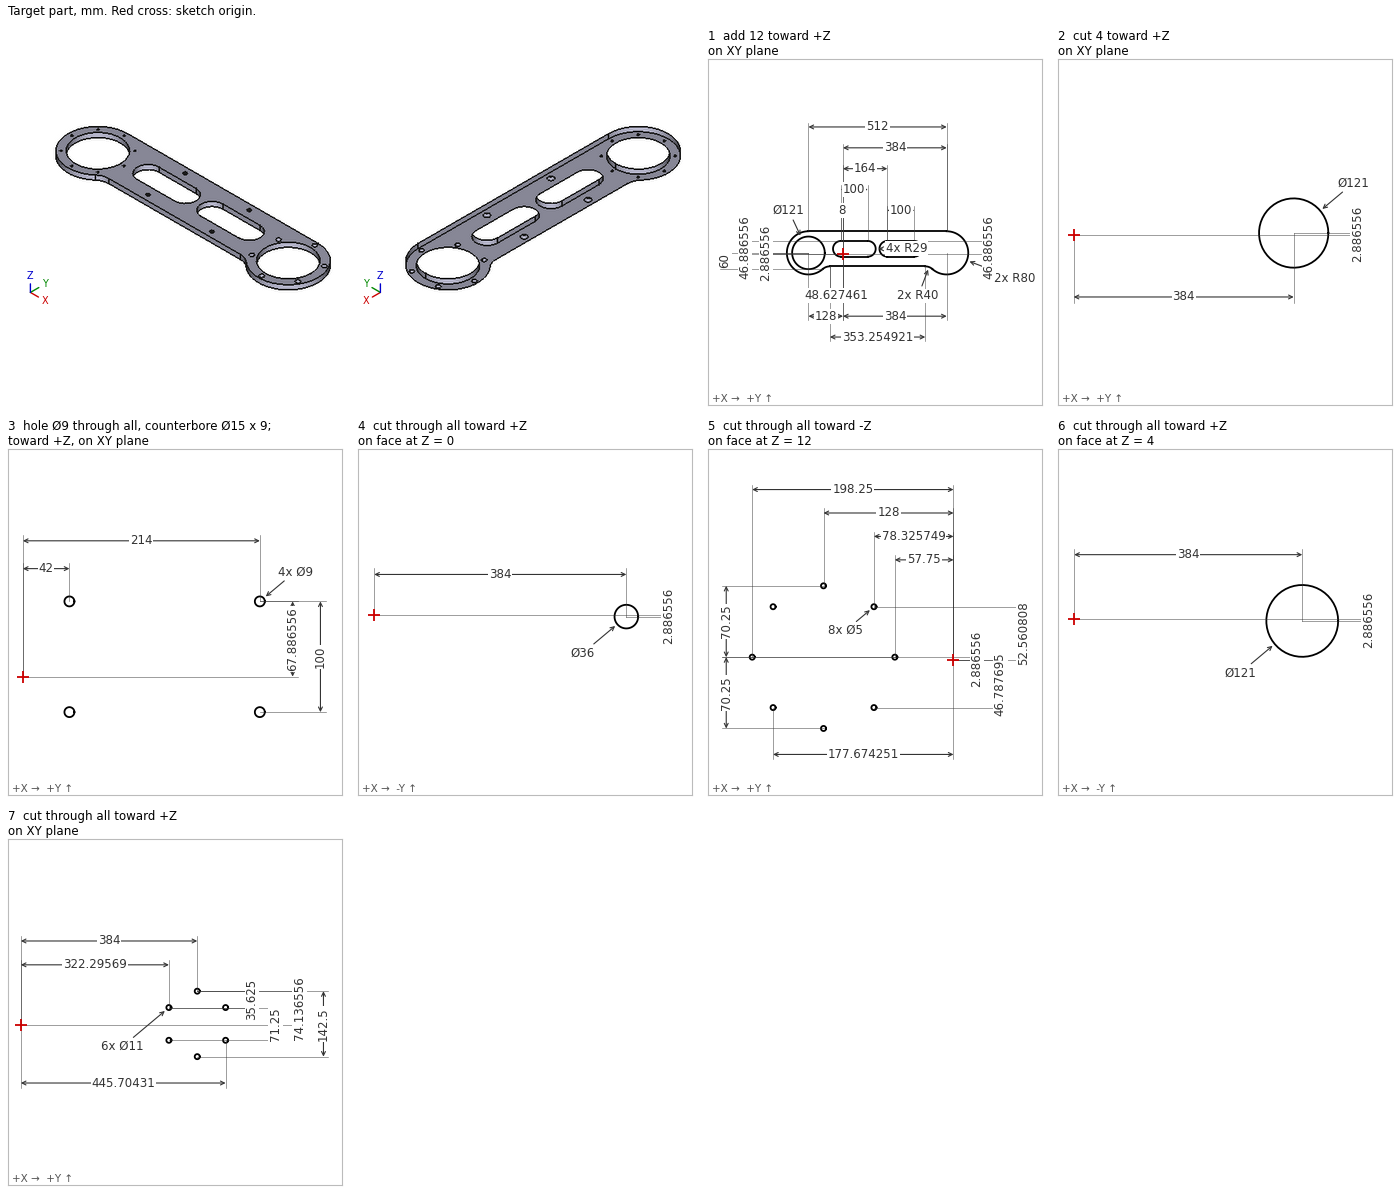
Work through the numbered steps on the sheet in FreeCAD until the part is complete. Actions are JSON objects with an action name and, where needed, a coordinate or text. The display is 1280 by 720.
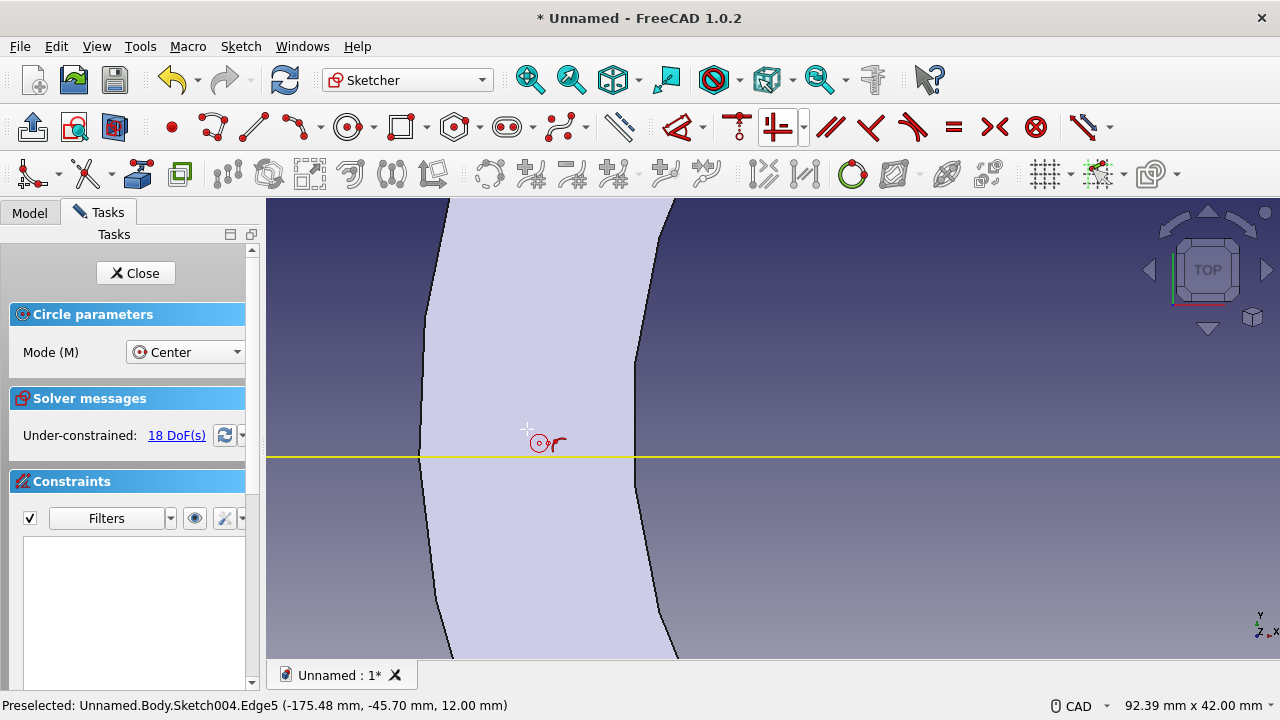
{"action": "left_click", "coordinate": [525, 425]}
{"action": "left_click", "coordinate": [545, 406]}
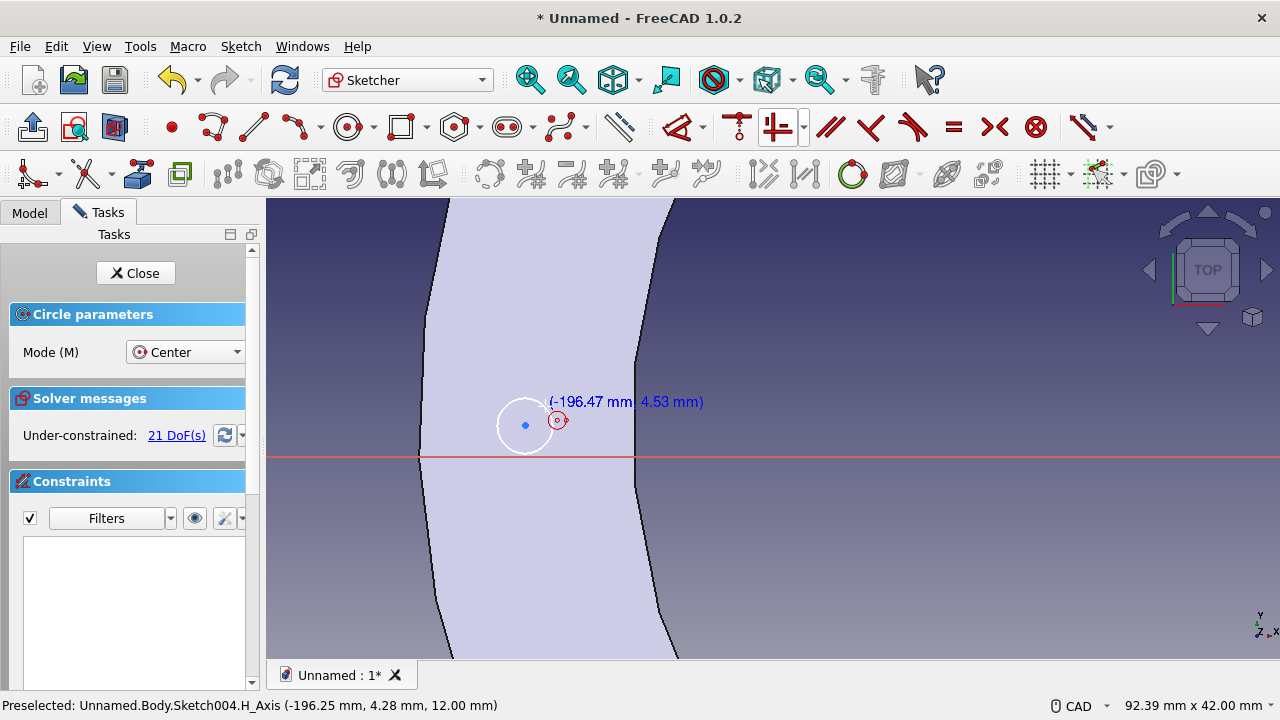
{"action": "scroll", "coordinate": [527, 429], "scroll_direction": "down", "scroll_amount": 9}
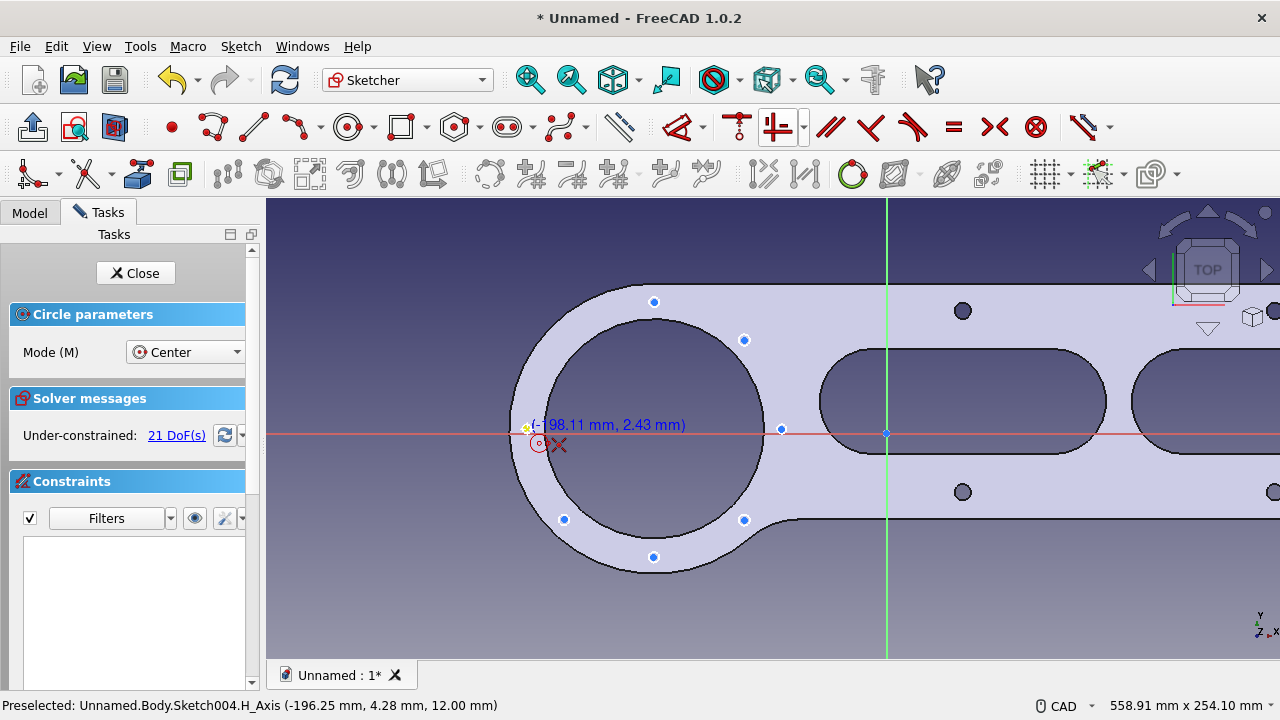
{"action": "scroll", "coordinate": [564, 339], "scroll_direction": "up", "scroll_amount": 9}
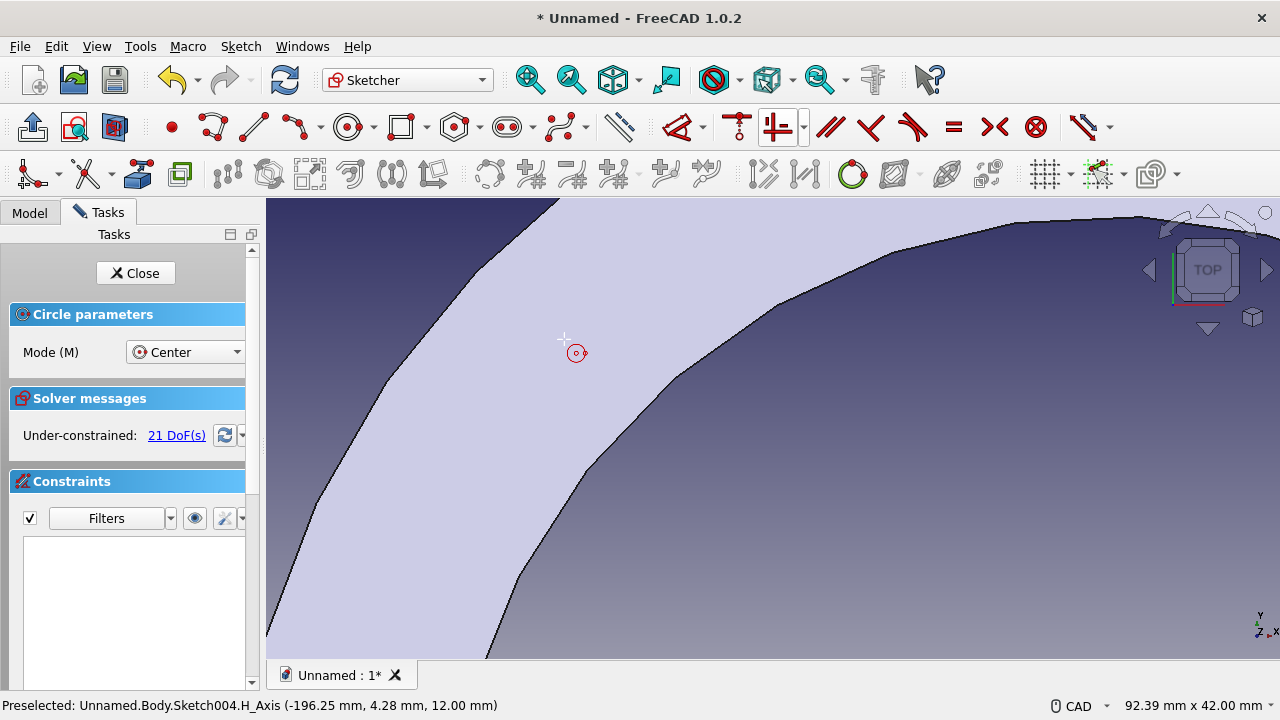
{"action": "scroll", "coordinate": [564, 339], "scroll_direction": "down", "scroll_amount": 9}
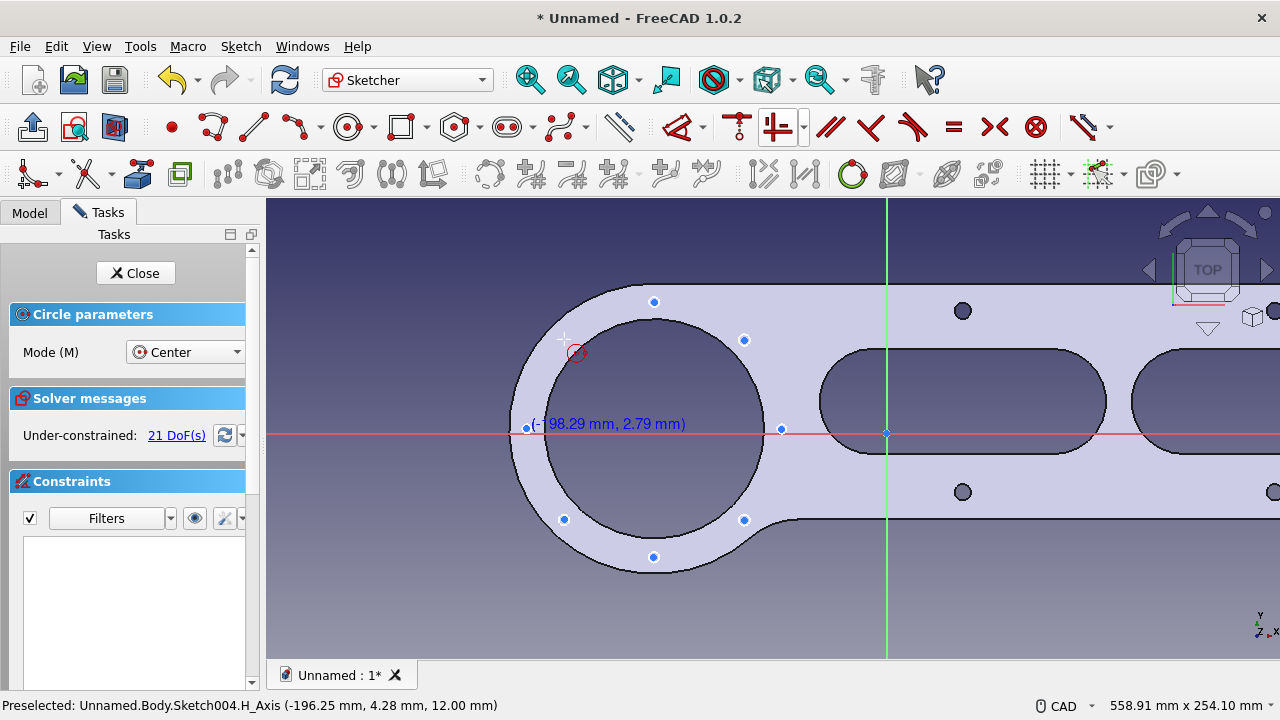
{"action": "left_click", "coordinate": [564, 339]}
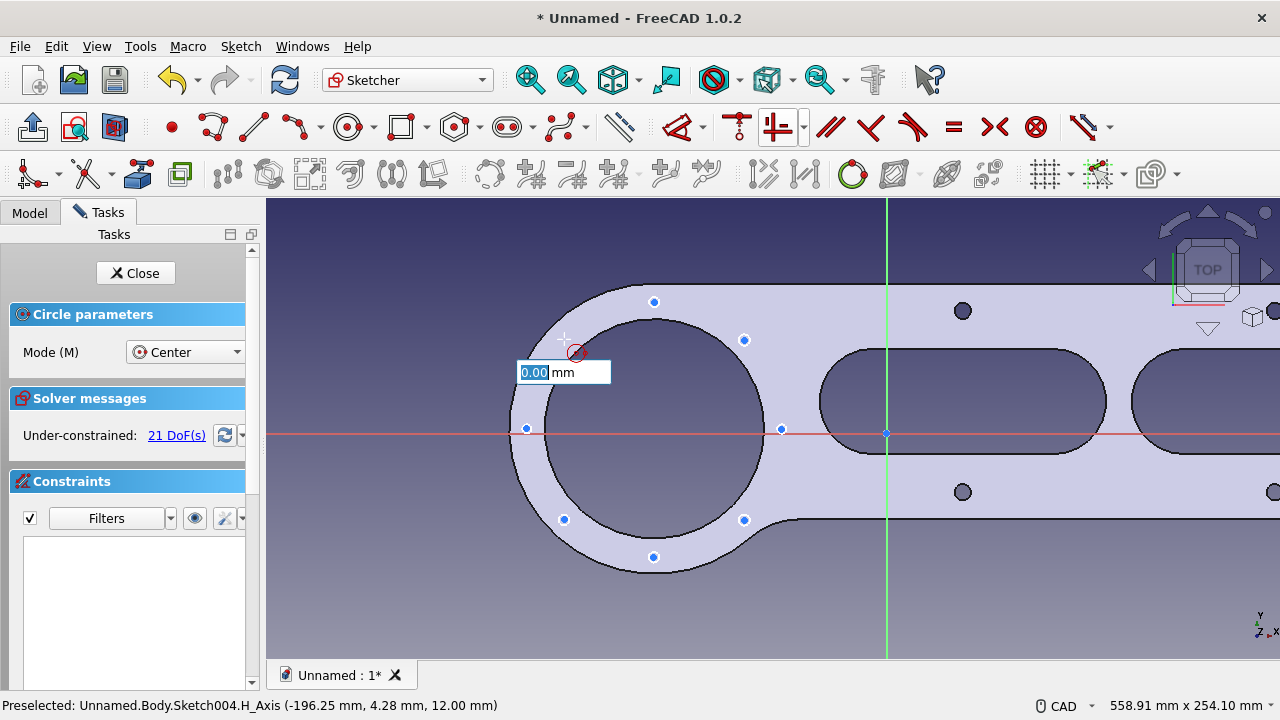
{"action": "scroll", "coordinate": [567, 335], "scroll_direction": "up", "scroll_amount": 7}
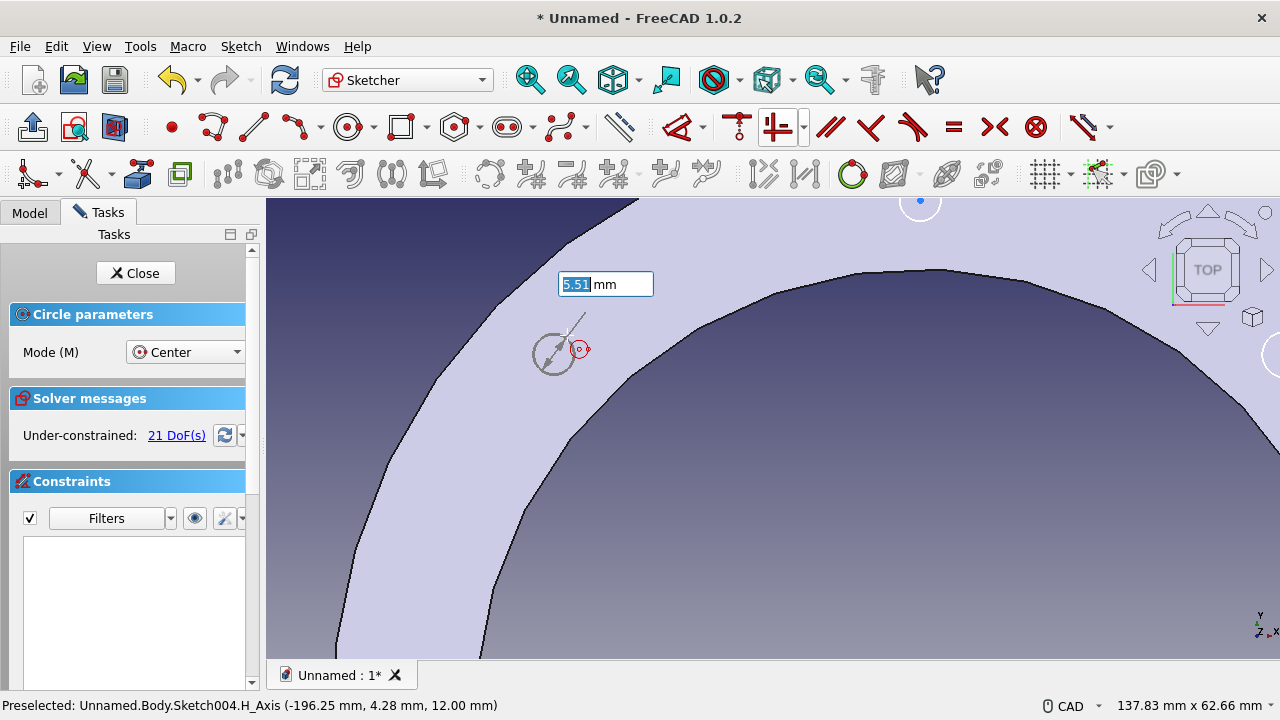
{"action": "left_click", "coordinate": [568, 336]}
{"action": "key", "text": "Escape"}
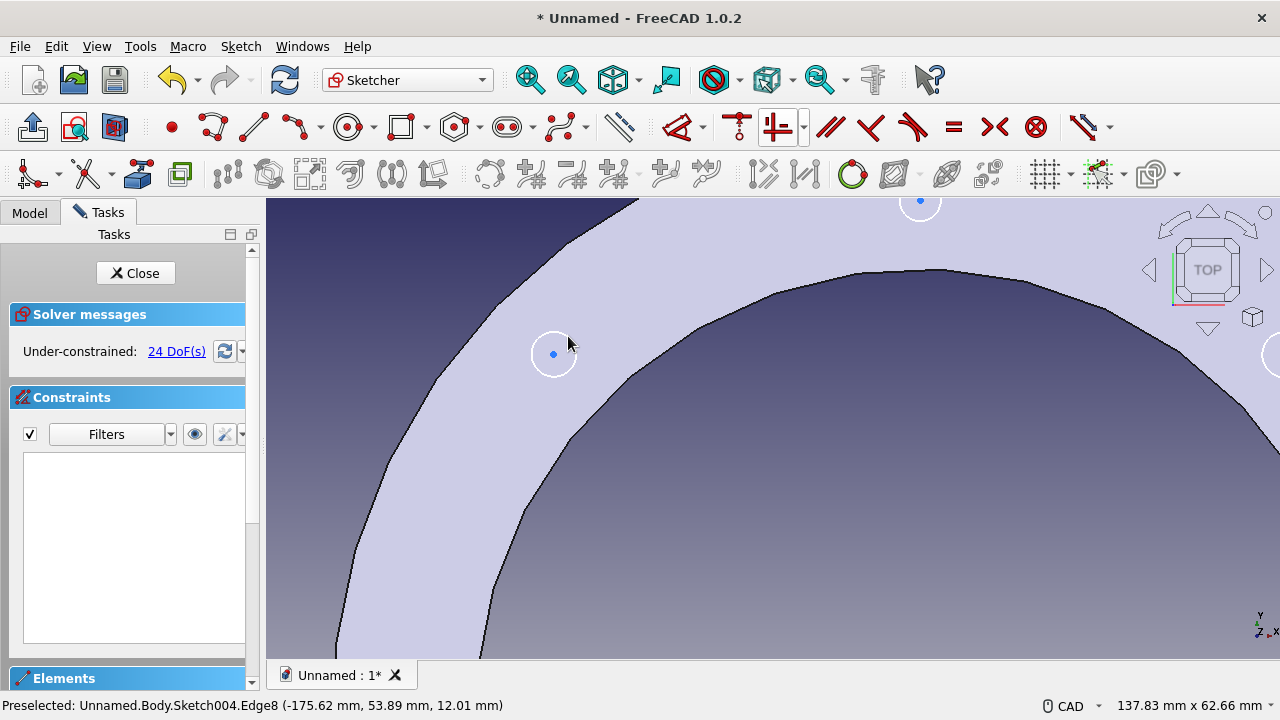
{"action": "scroll", "coordinate": [567, 335], "scroll_direction": "down", "scroll_amount": 7}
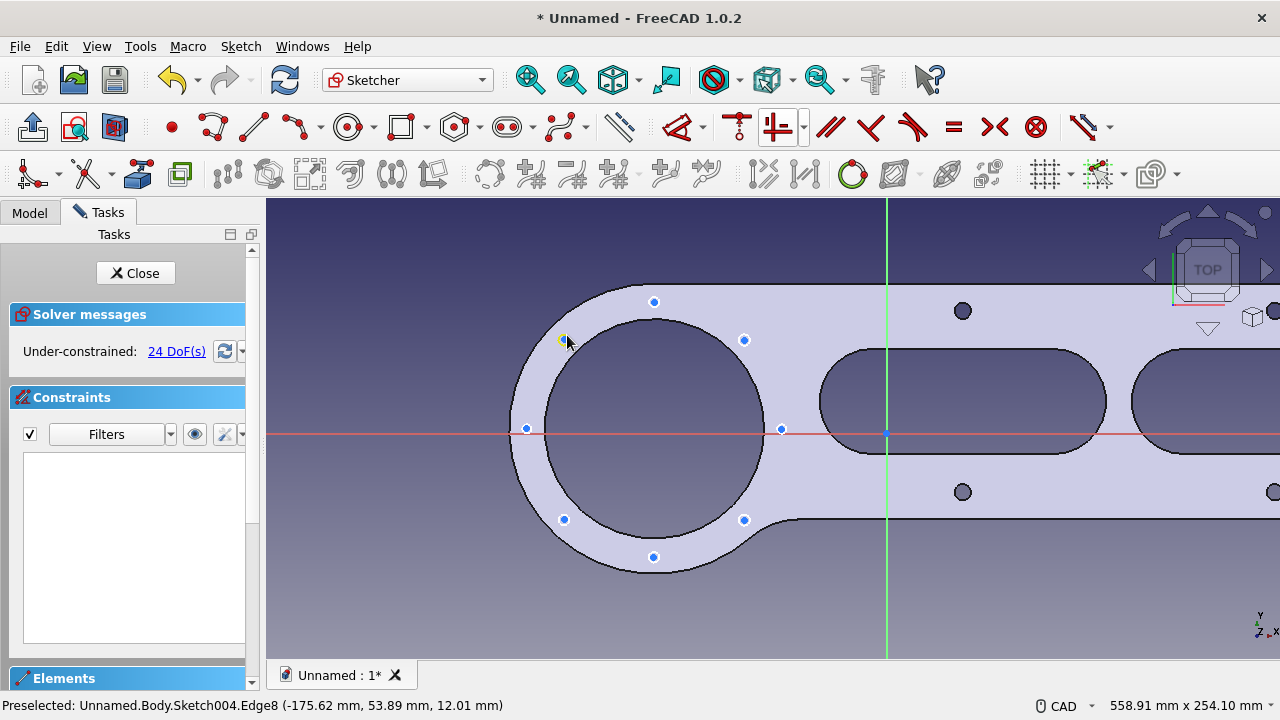
{"action": "scroll", "coordinate": [748, 336], "scroll_direction": "up", "scroll_amount": 5}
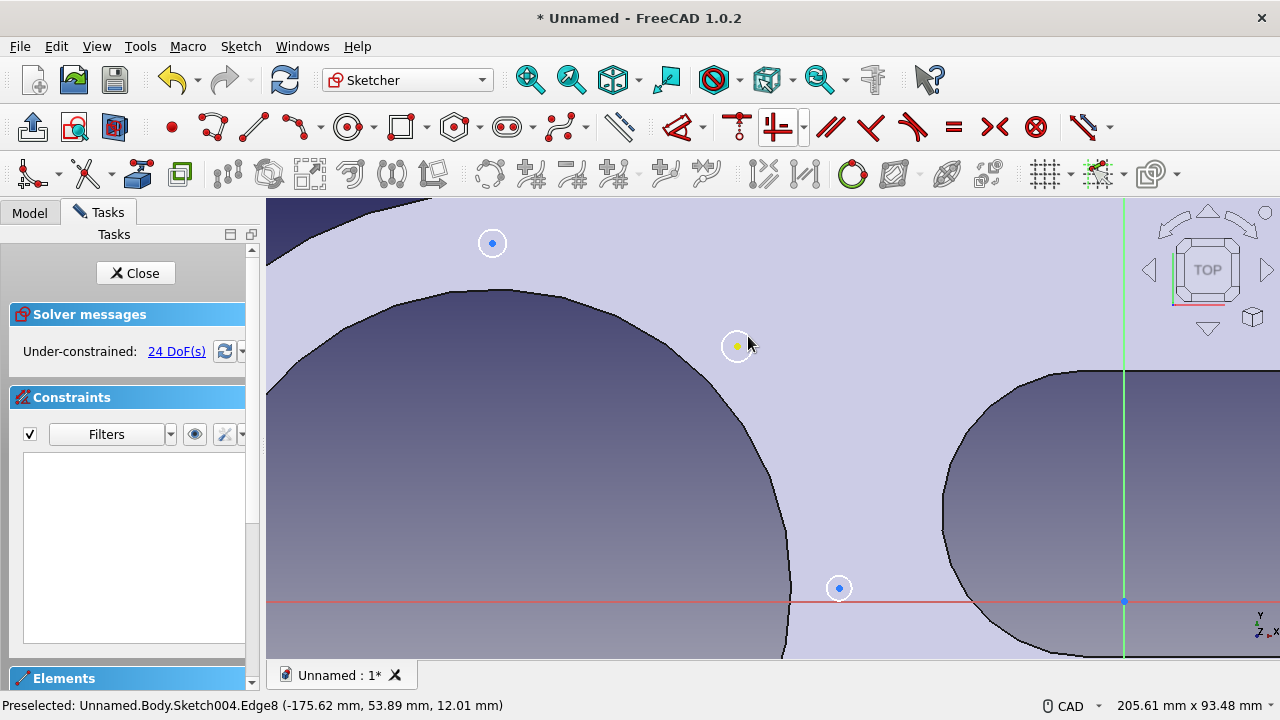
{"action": "left_click", "coordinate": [748, 336]}